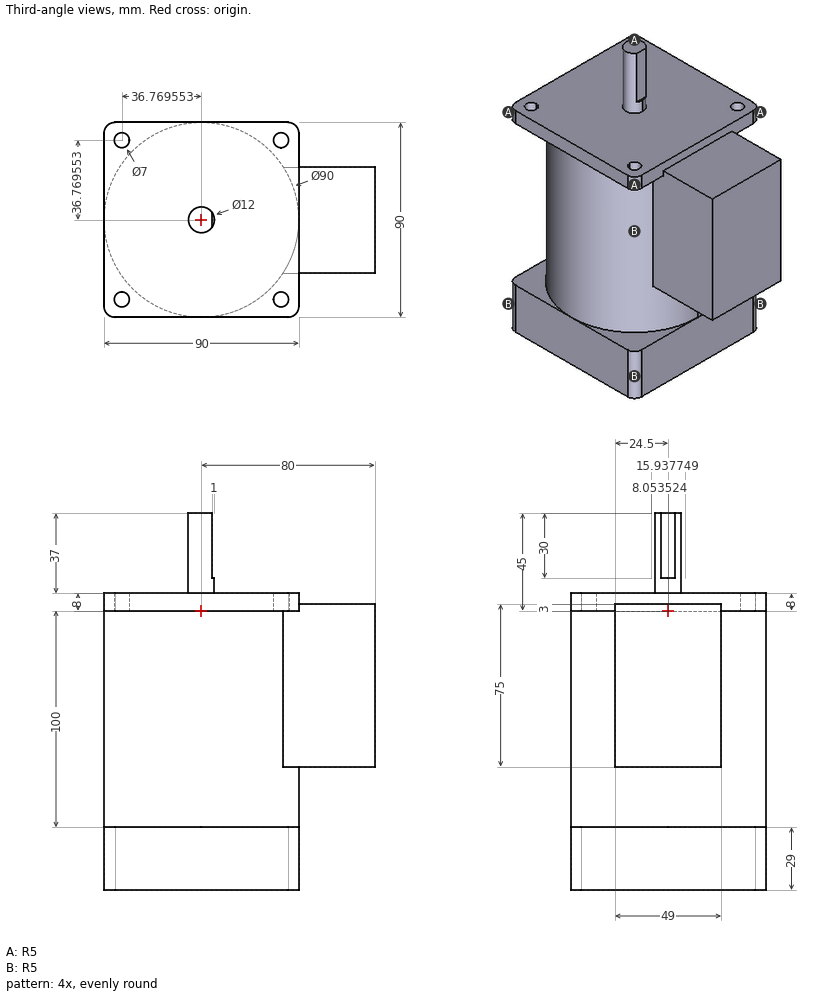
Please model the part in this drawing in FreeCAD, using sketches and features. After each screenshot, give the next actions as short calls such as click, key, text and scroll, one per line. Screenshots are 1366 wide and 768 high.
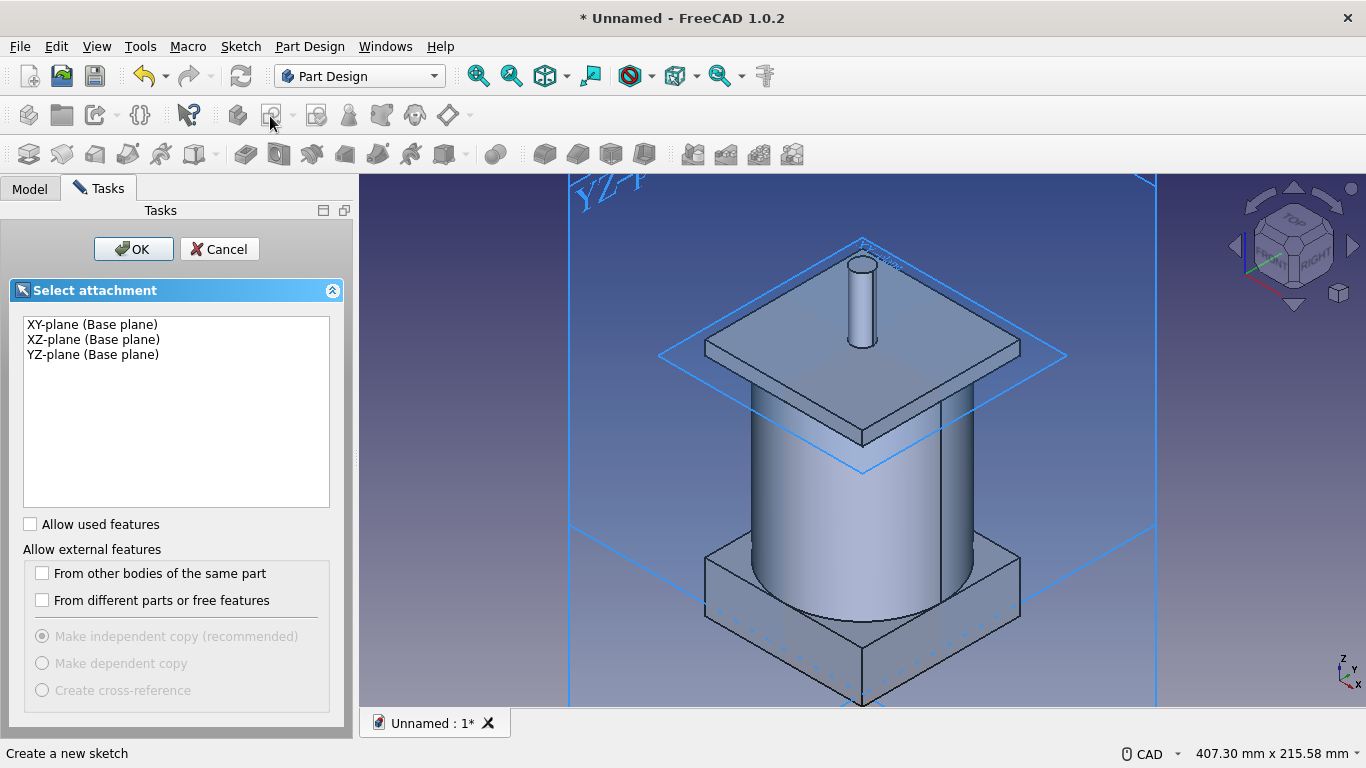
click(84, 354)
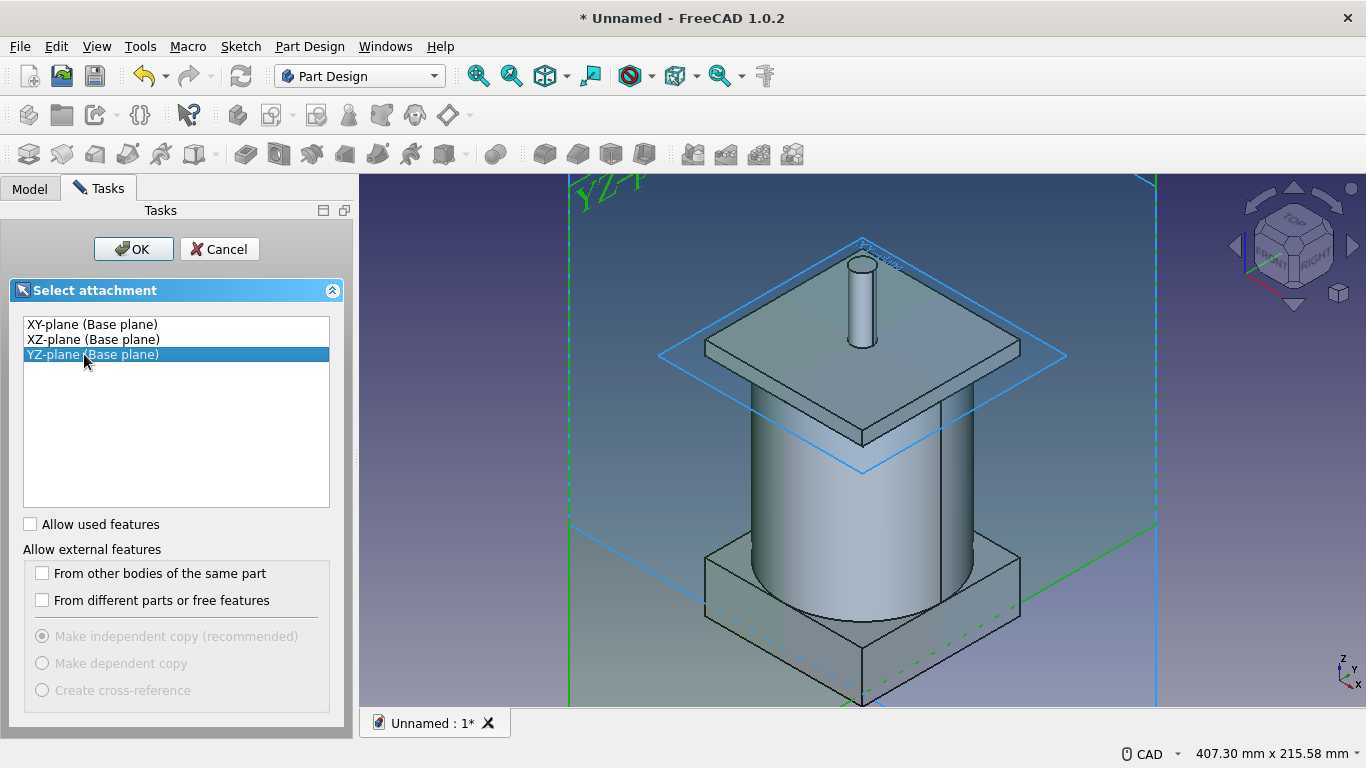
click(134, 249)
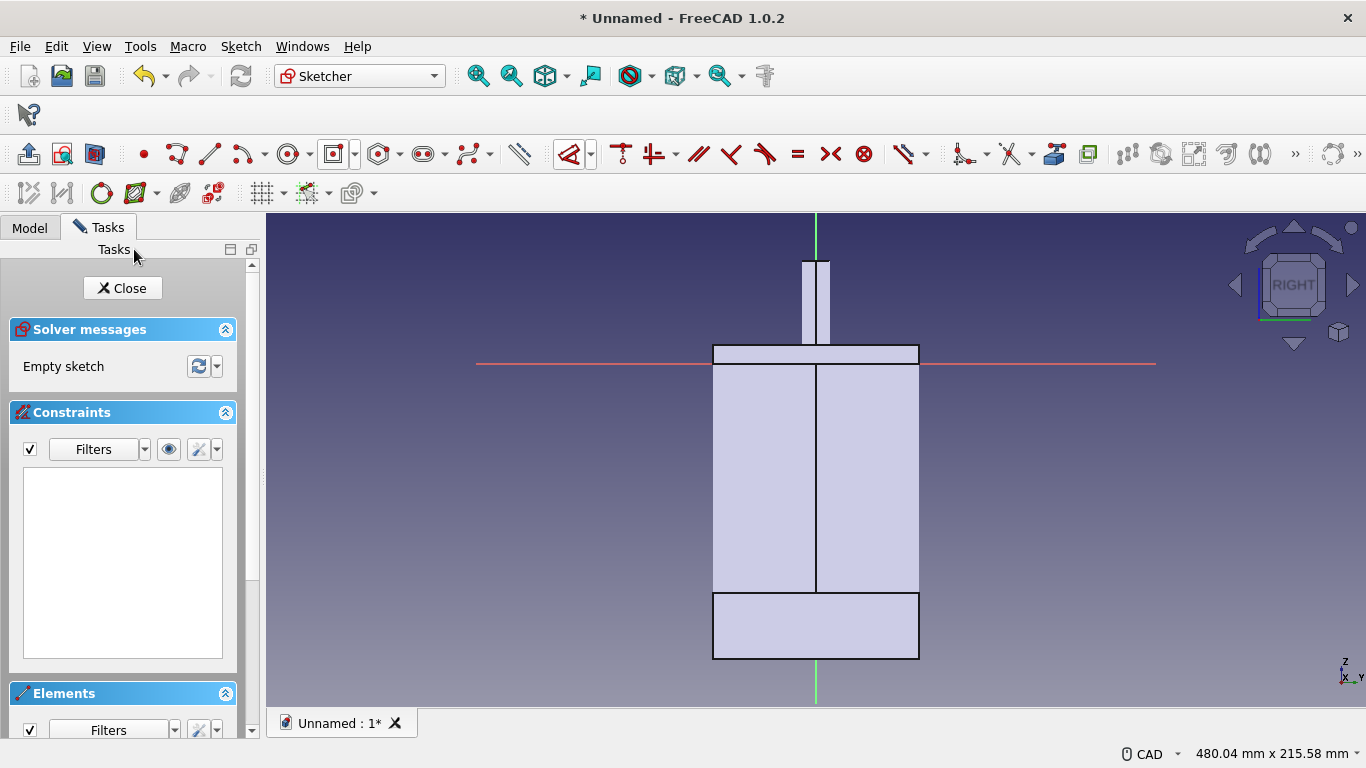
click(95, 154)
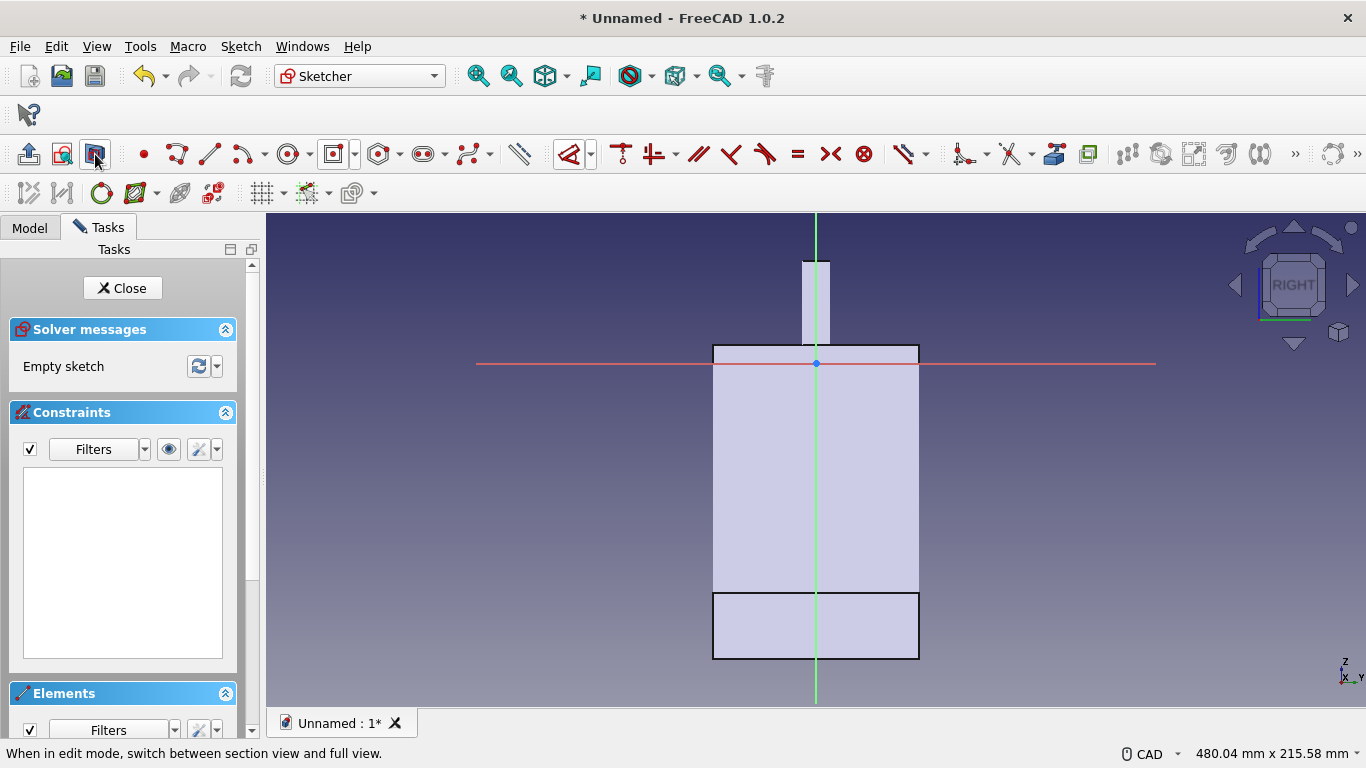
scroll(899, 422, up, 3)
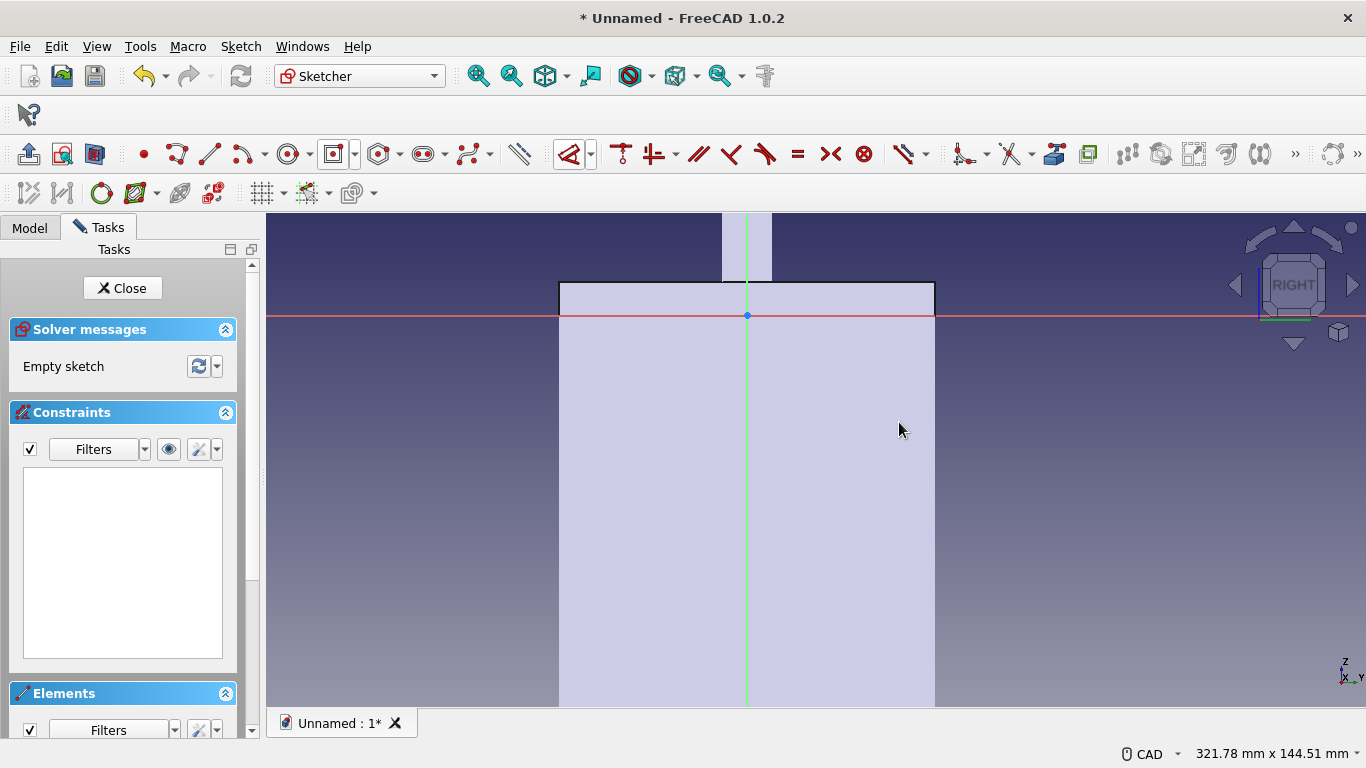
click(354, 154)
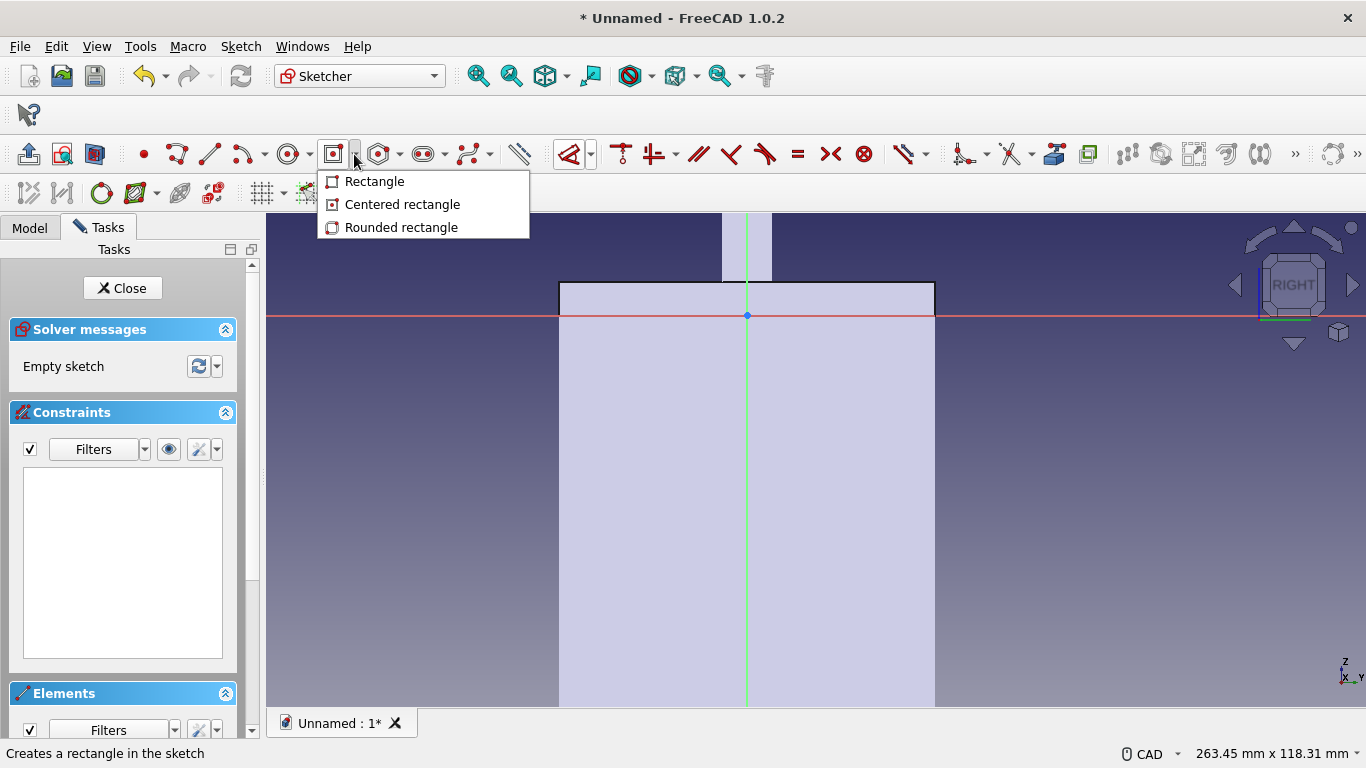
click(424, 182)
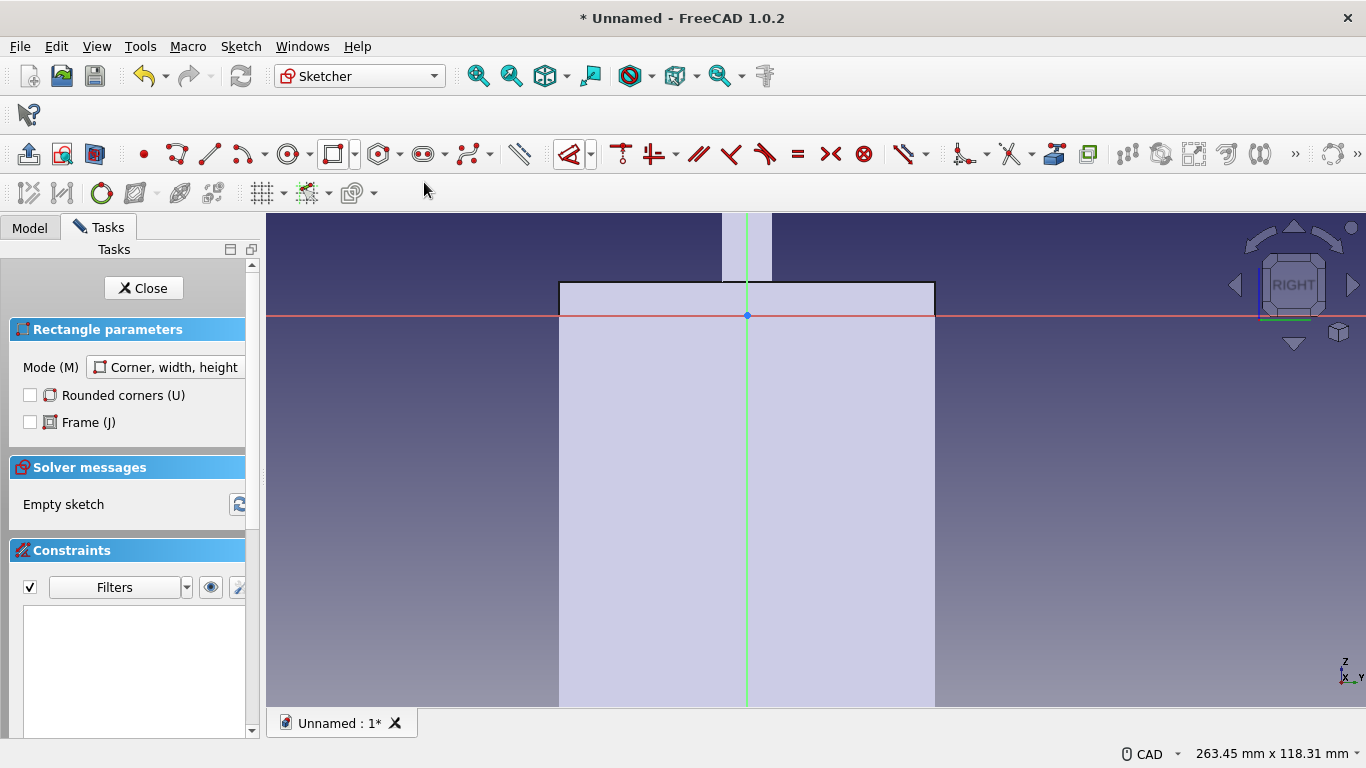
scroll(645, 303, up, 2)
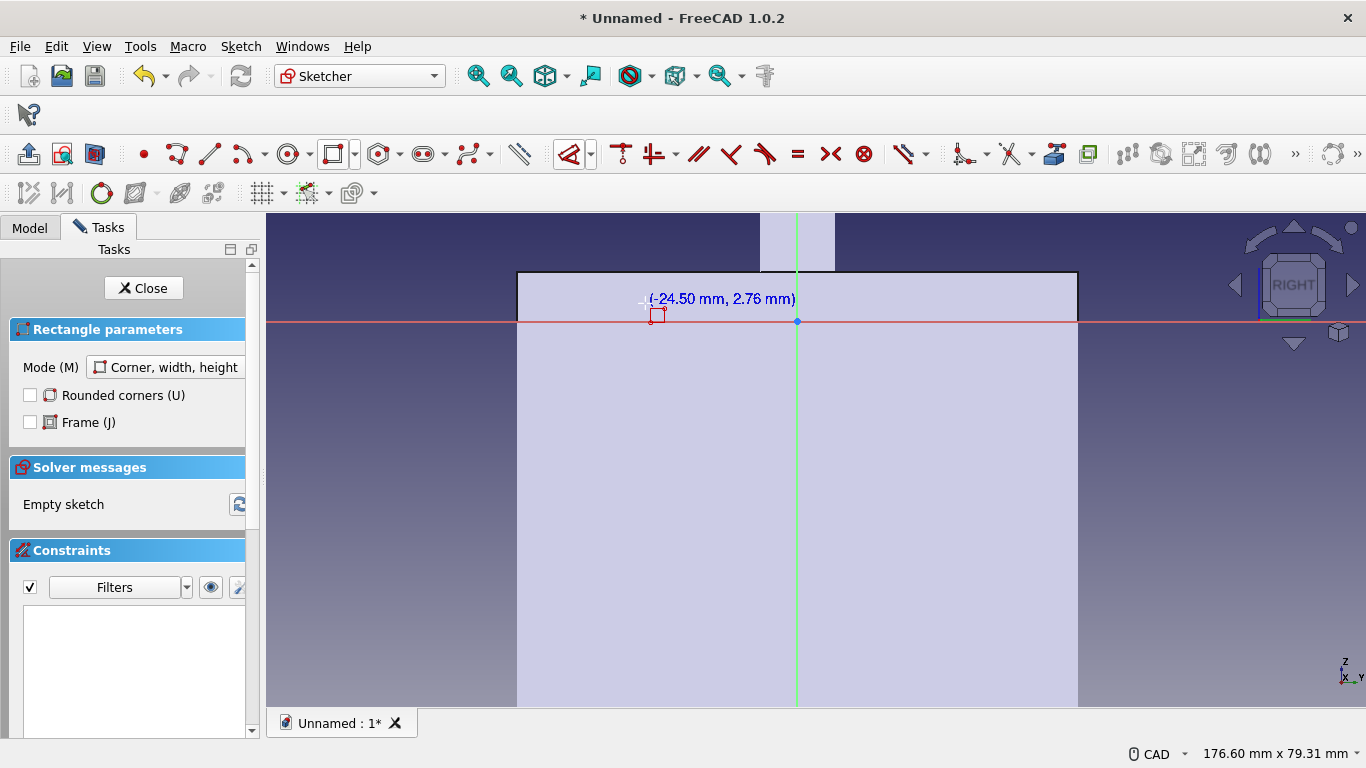
click(645, 303)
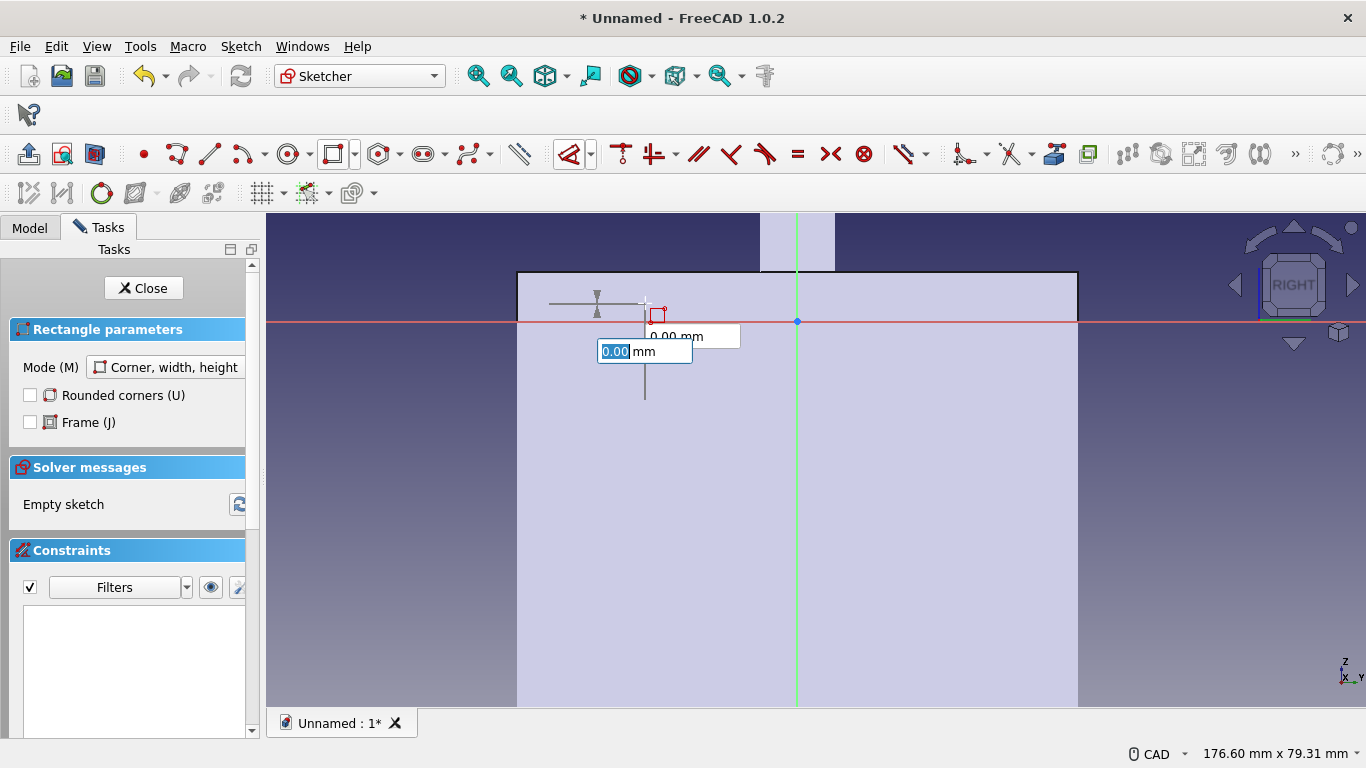
scroll(646, 304, down, 2)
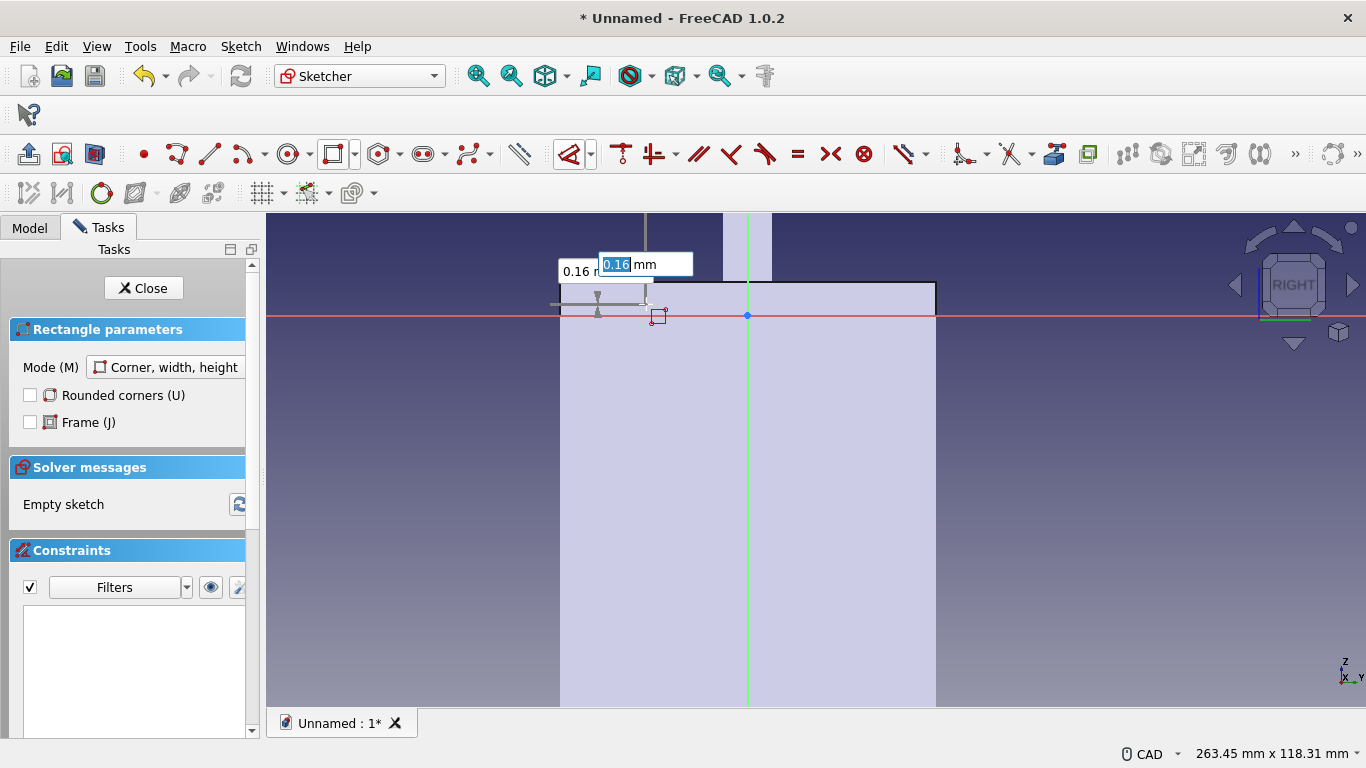
click(850, 616)
key(Escape)